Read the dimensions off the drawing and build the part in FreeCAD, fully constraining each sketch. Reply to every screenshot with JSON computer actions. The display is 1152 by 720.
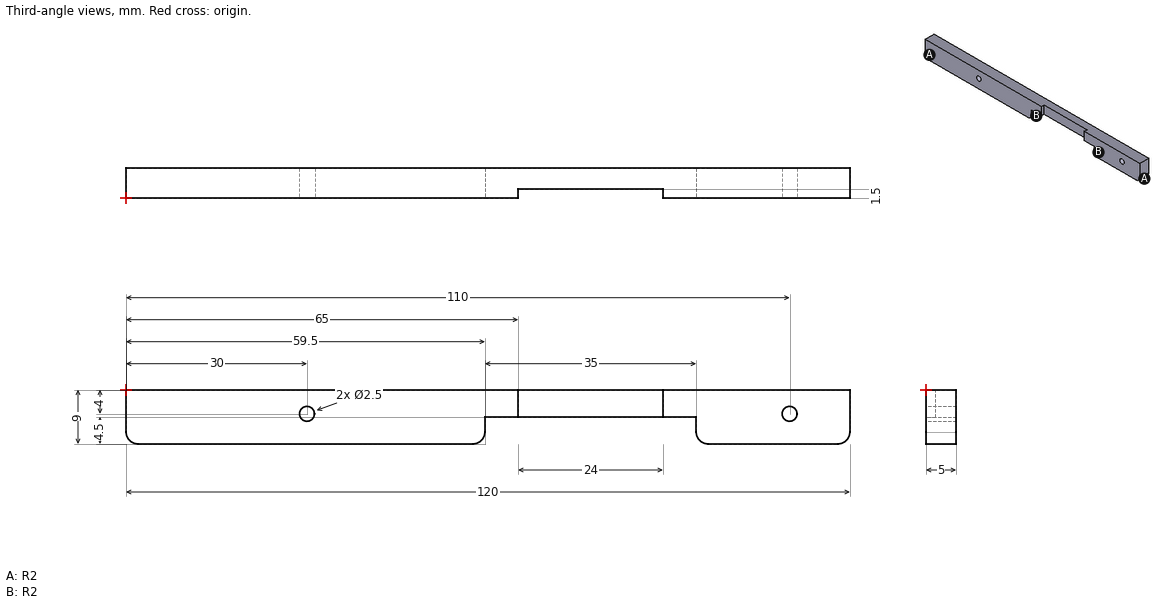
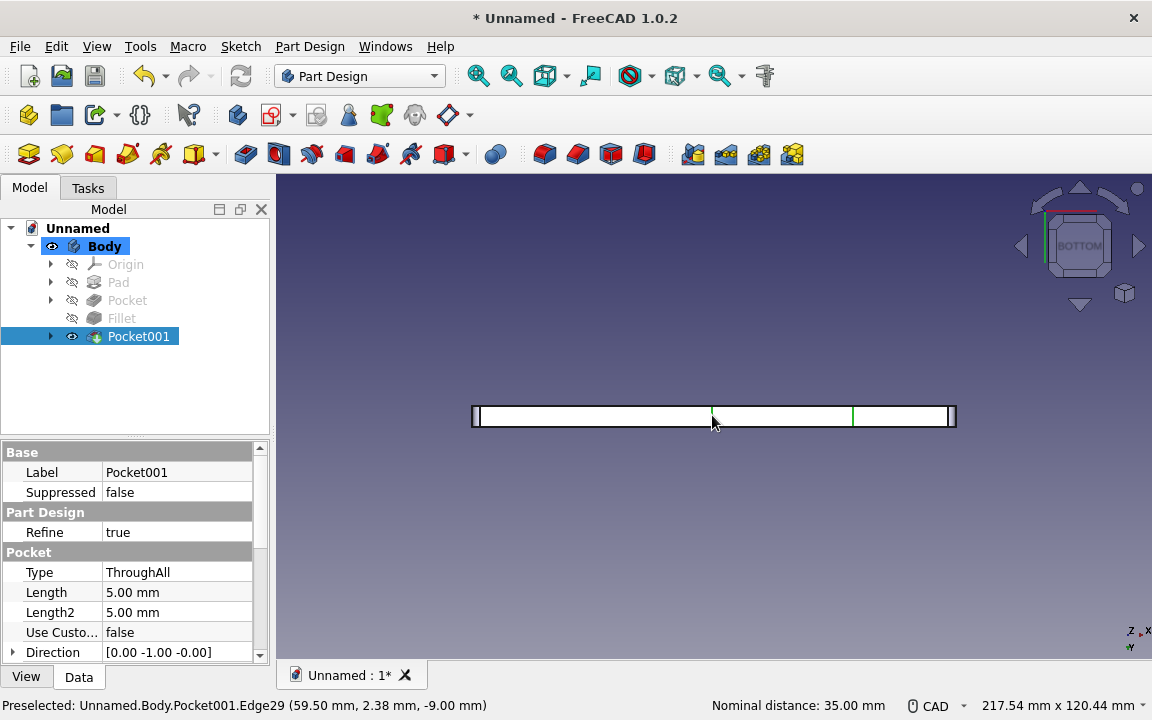
{"action": "left_click", "coordinate": [545, 154]}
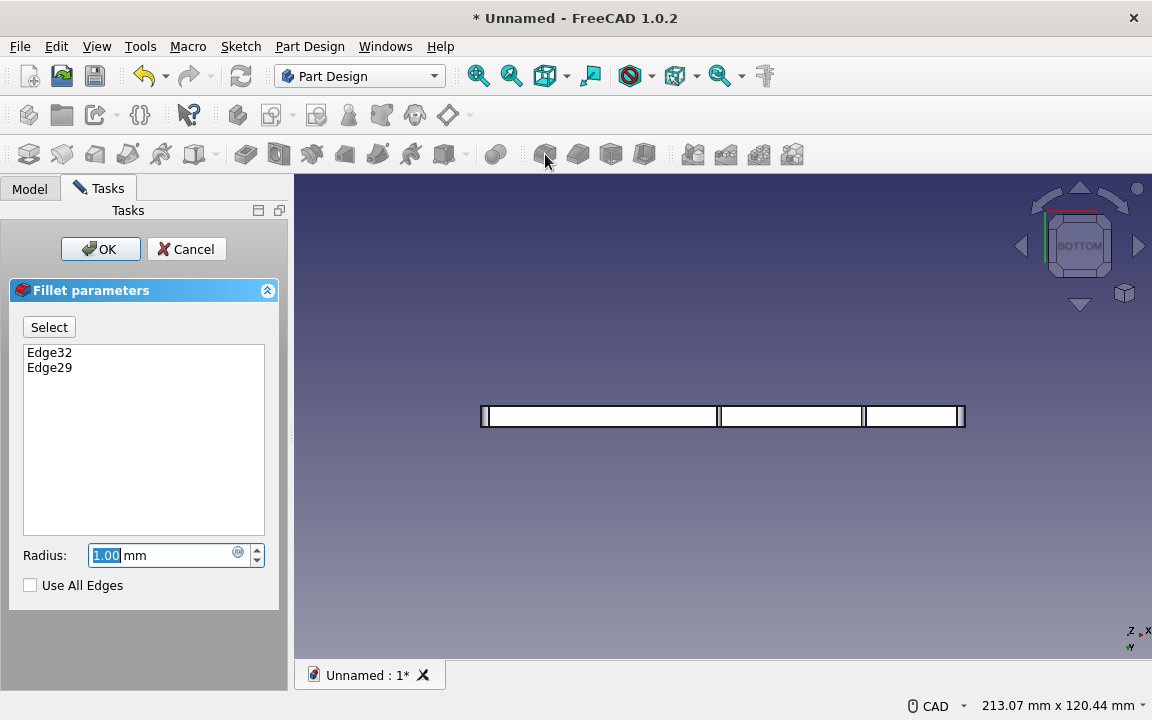
{"action": "type", "text": "2"}
{"action": "key", "text": "Tab"}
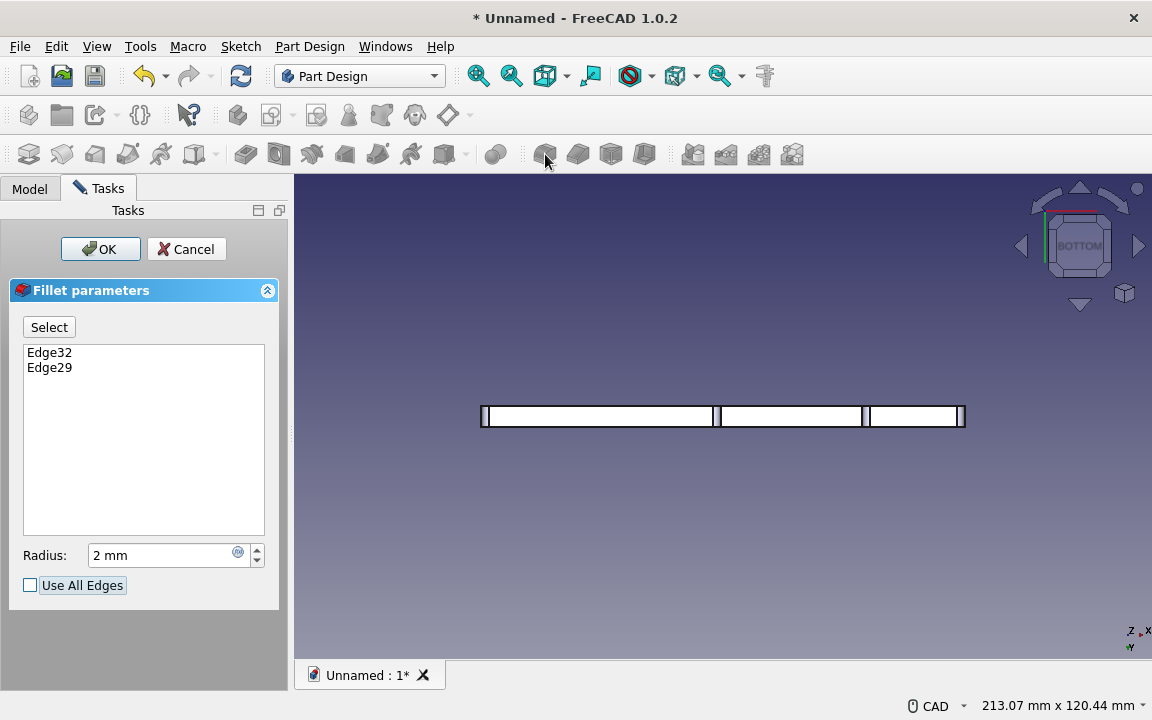
{"action": "left_click", "coordinate": [101, 249]}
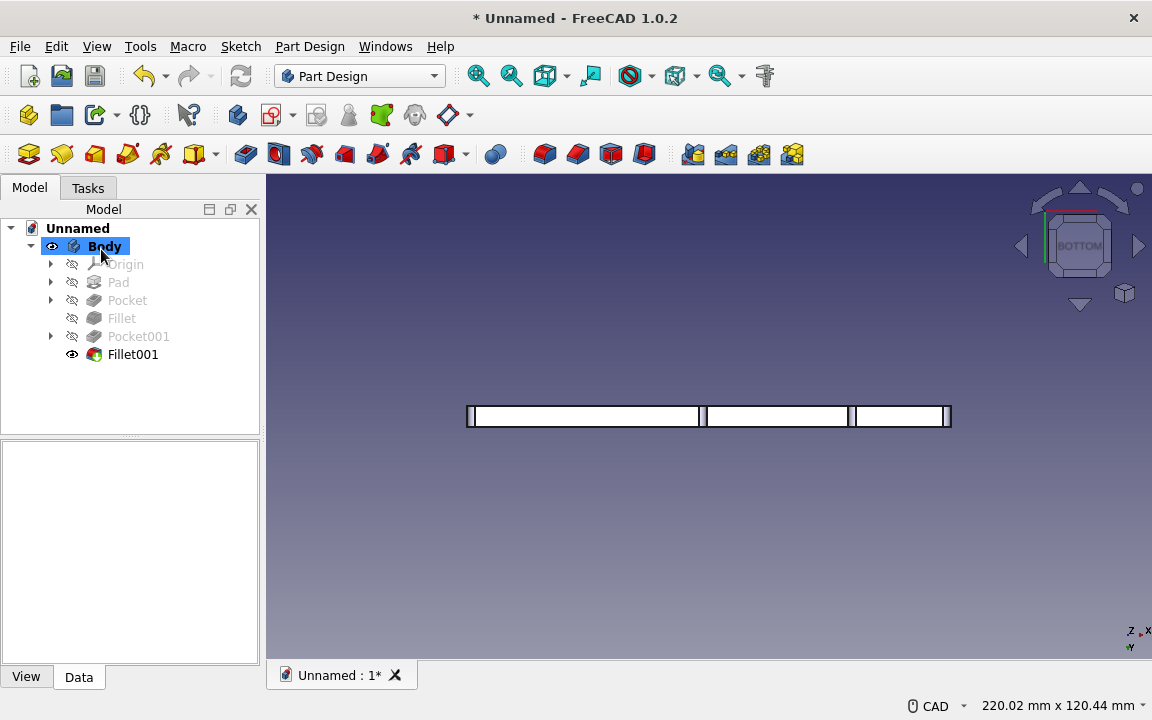
{"action": "left_click", "coordinate": [270, 116]}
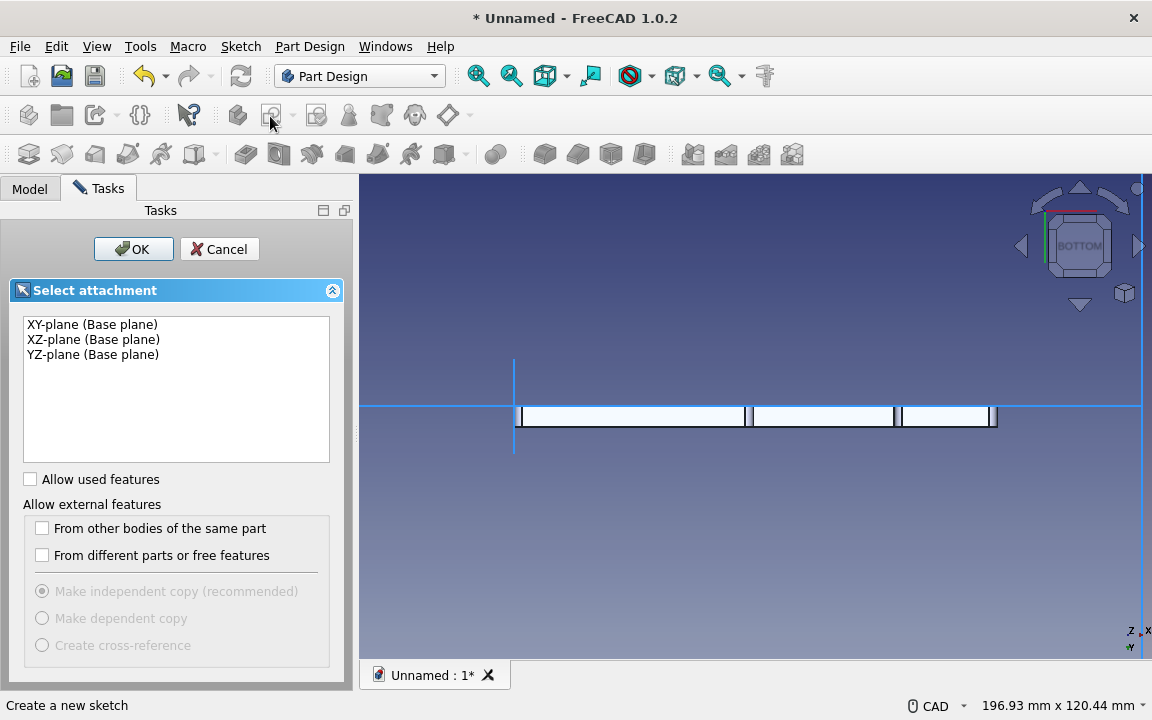
{"action": "left_click", "coordinate": [84, 340]}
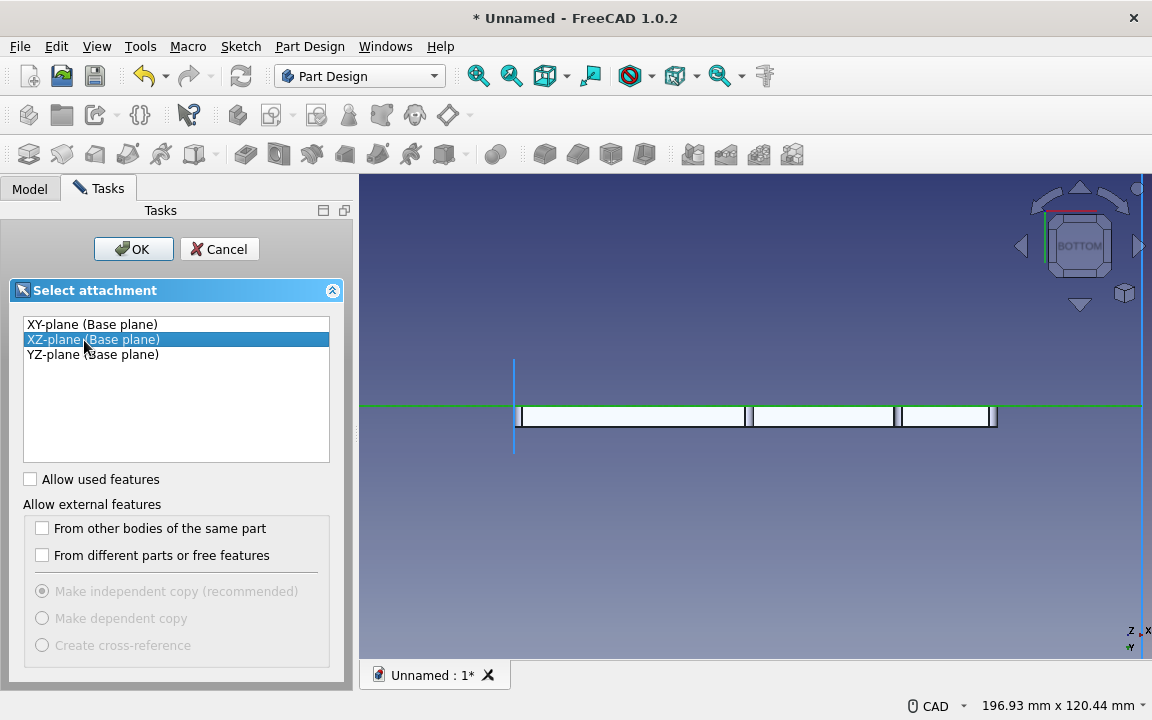
{"action": "left_click", "coordinate": [134, 249]}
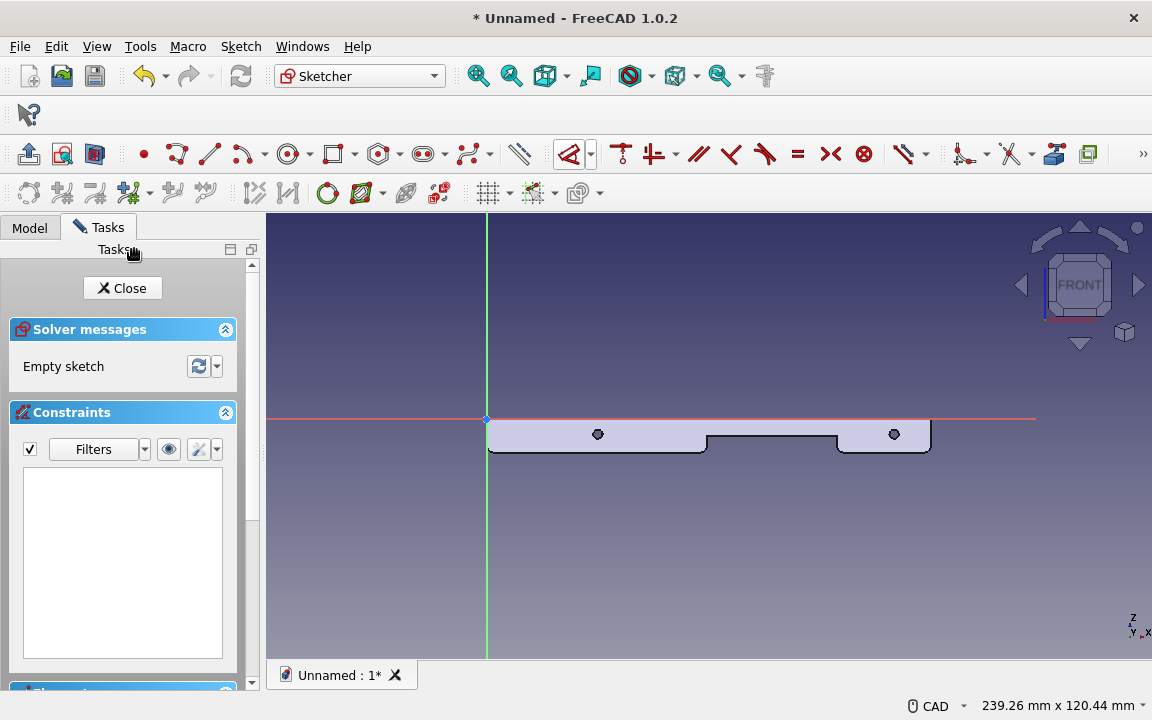
{"action": "scroll", "coordinate": [798, 436], "scroll_direction": "up", "scroll_amount": 9}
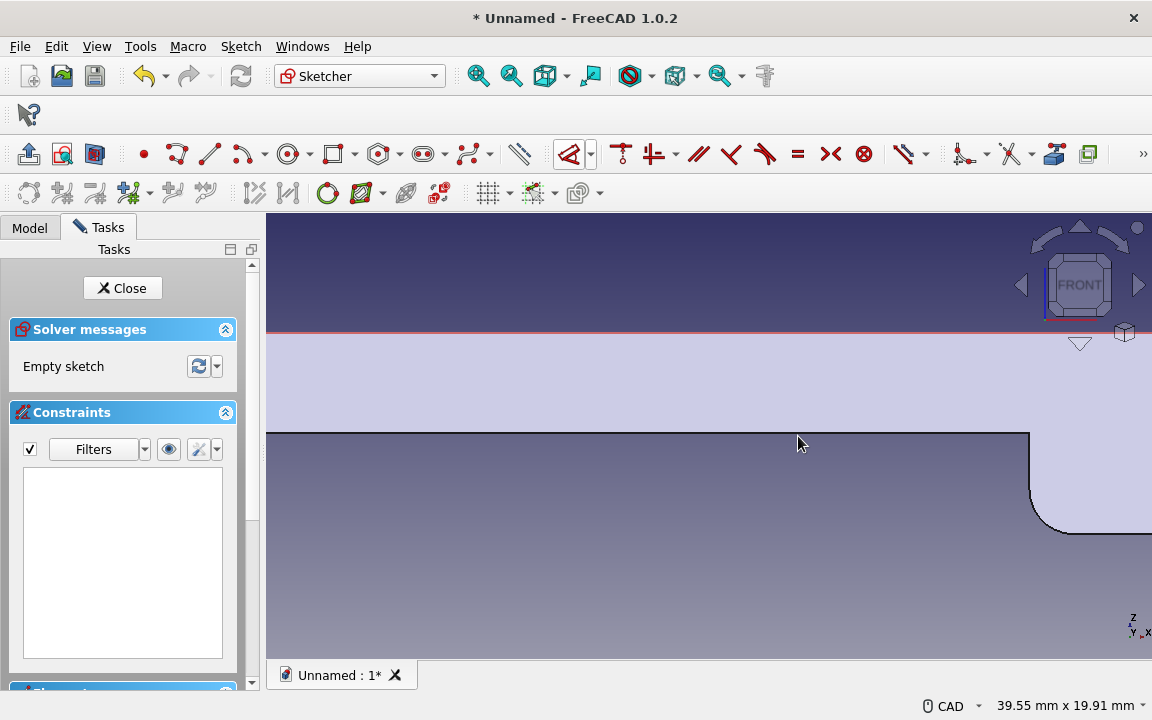
{"action": "key", "text": "g r"}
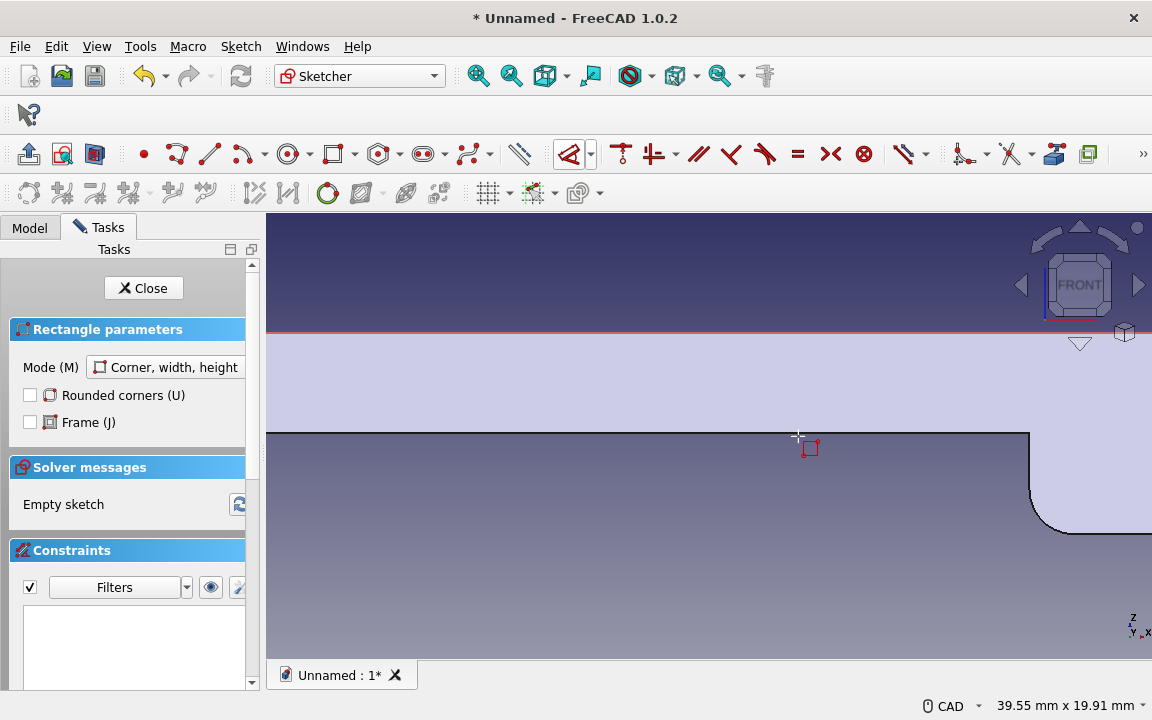
{"action": "left_click", "coordinate": [369, 333]}
{"action": "left_click", "coordinate": [906, 534]}
{"action": "key", "text": "Escape"}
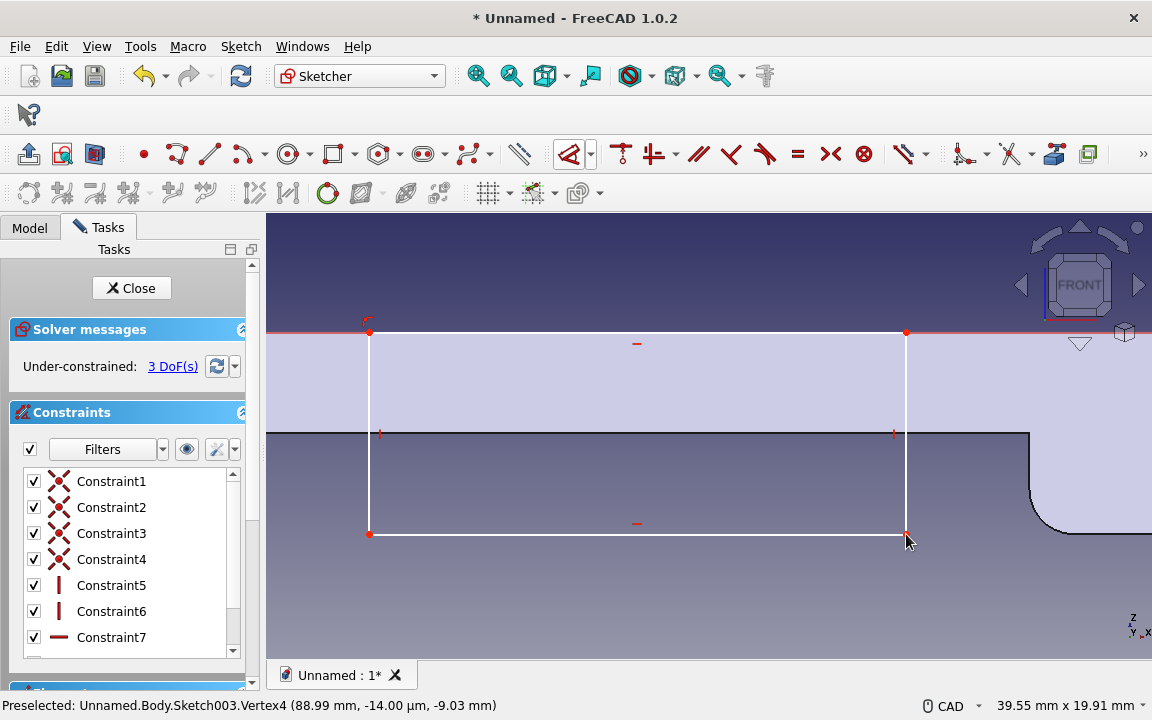
{"action": "key", "text": "d"}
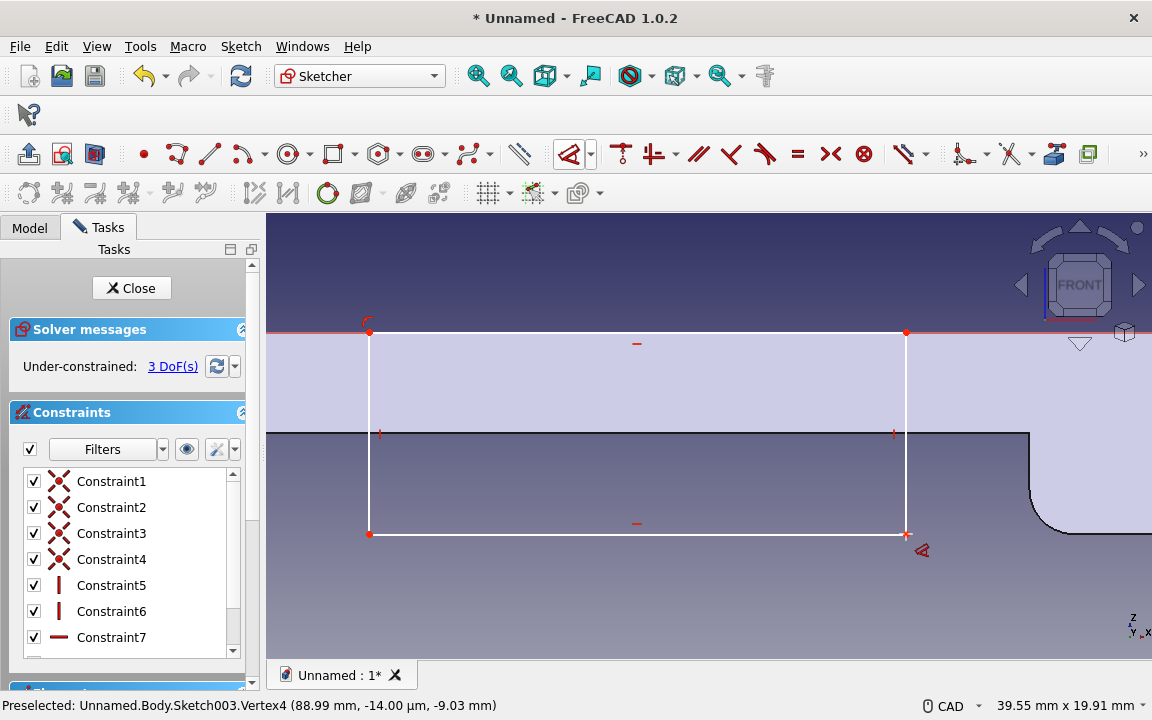
{"action": "left_click", "coordinate": [369, 393]}
{"action": "left_click", "coordinate": [335, 434]}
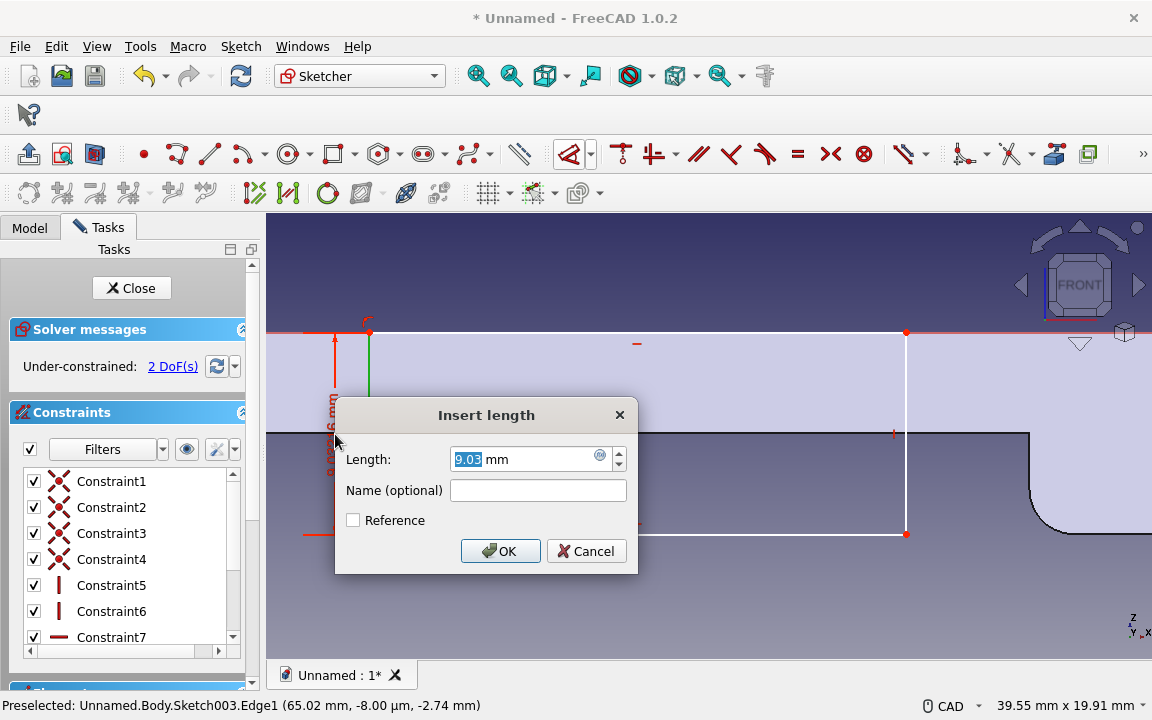
{"action": "type", "text": "9"}
{"action": "key", "text": "Return"}